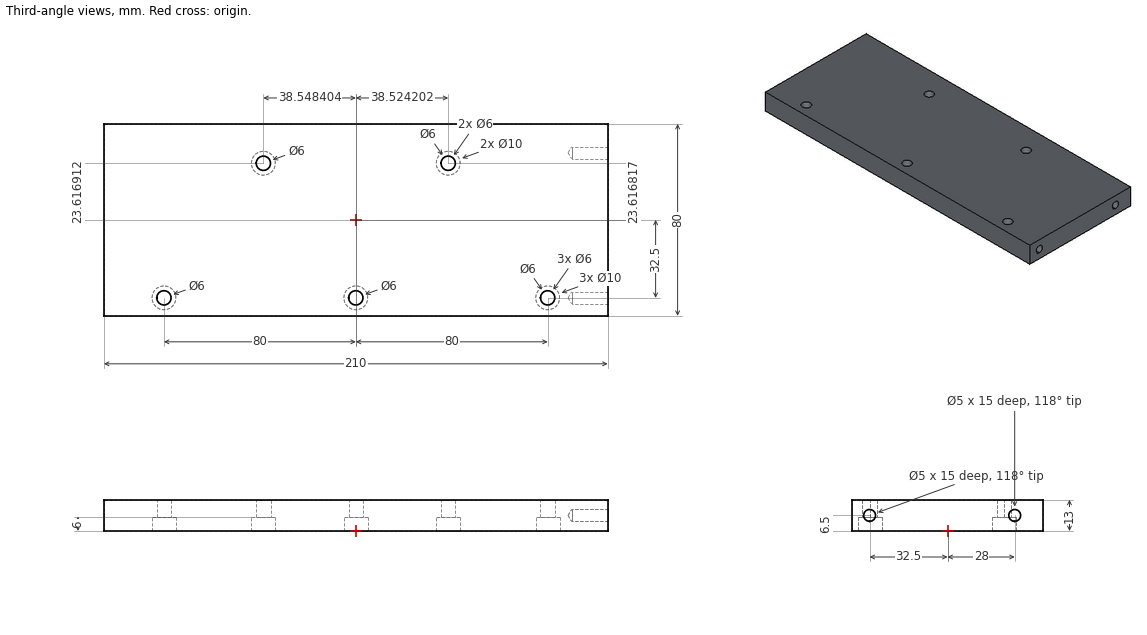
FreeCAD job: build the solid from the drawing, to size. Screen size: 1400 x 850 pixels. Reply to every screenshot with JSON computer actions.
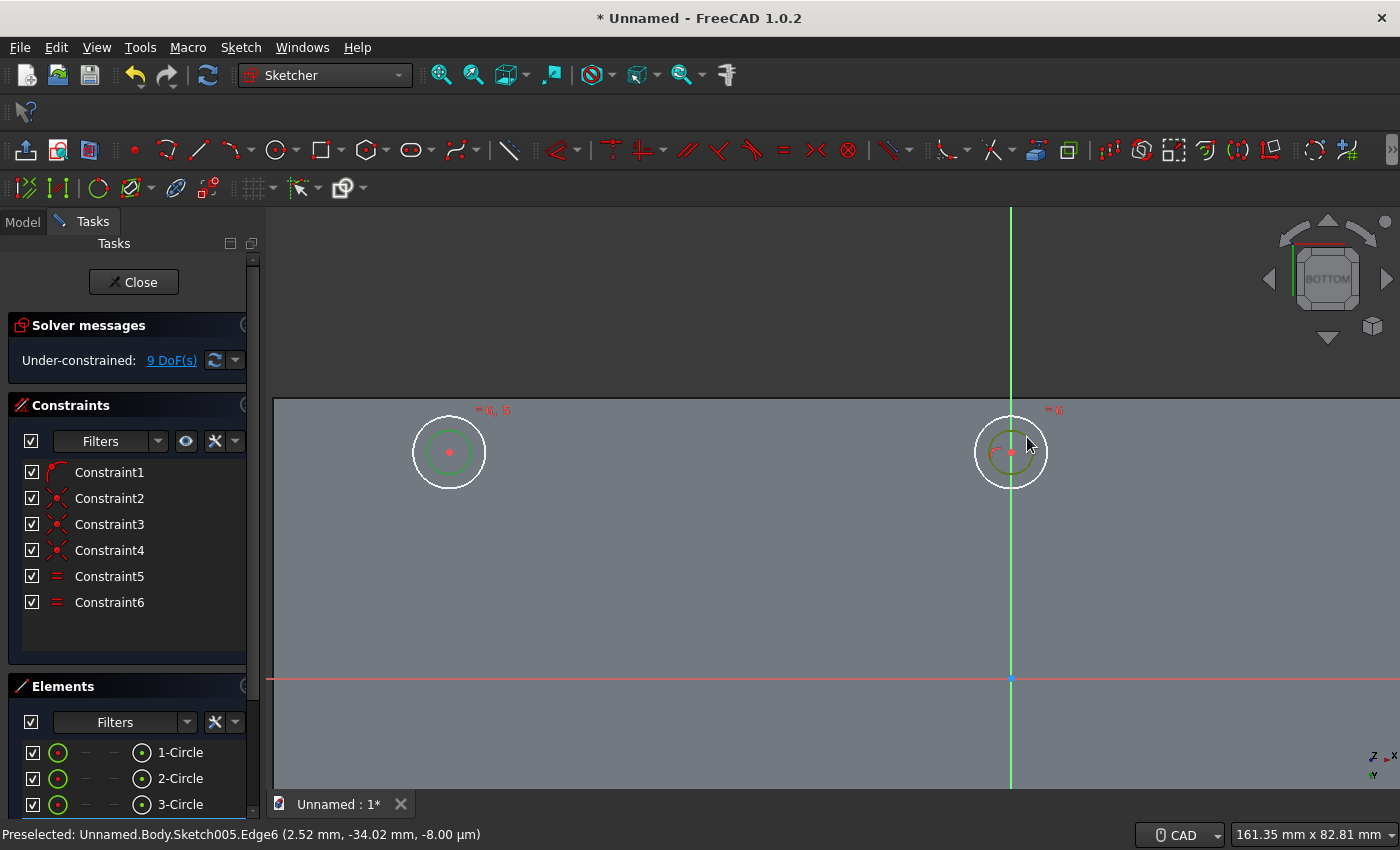
{"action": "left_click", "coordinate": [784, 150]}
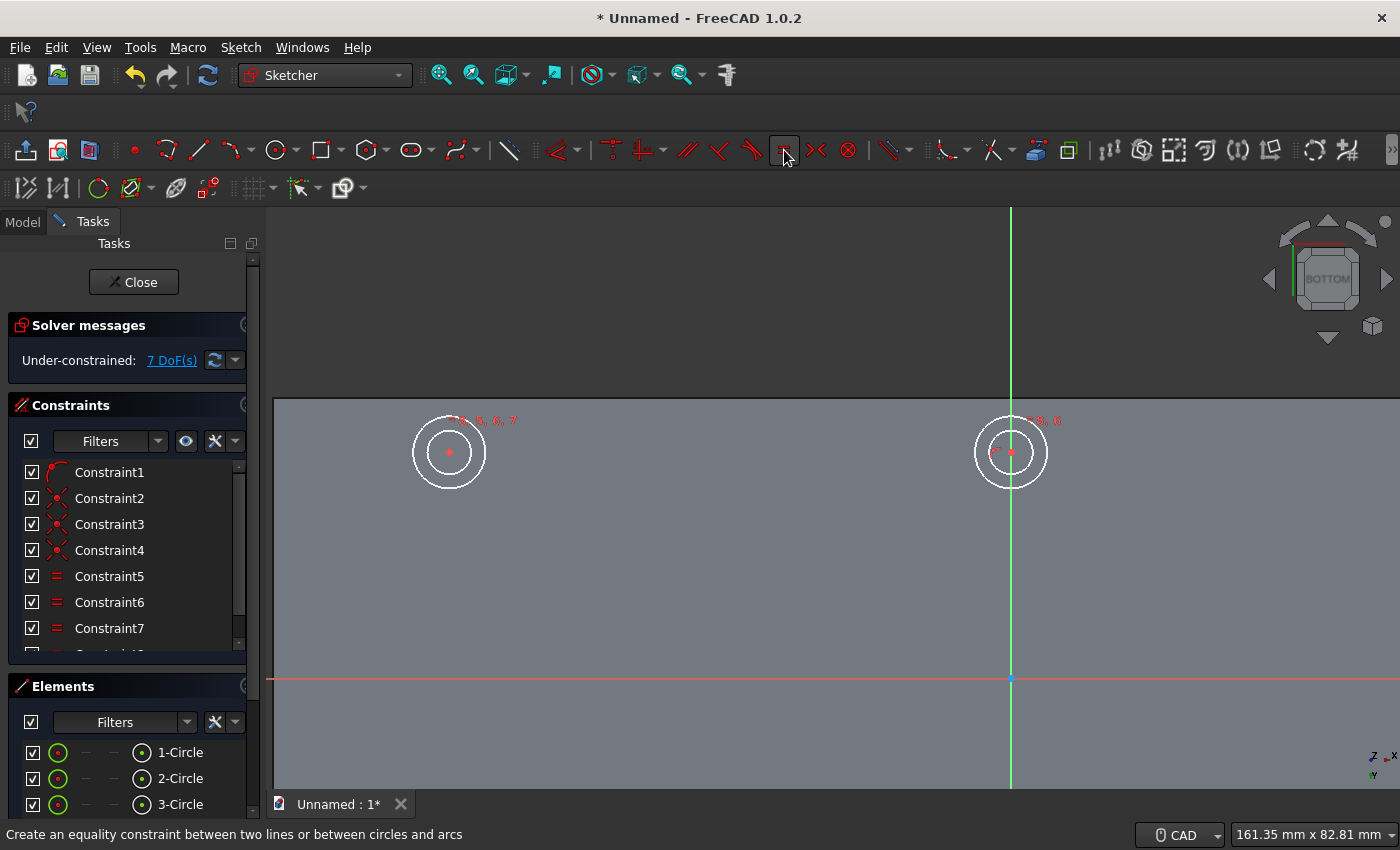
{"action": "scroll", "coordinate": [465, 438], "scroll_direction": "down", "scroll_amount": 3}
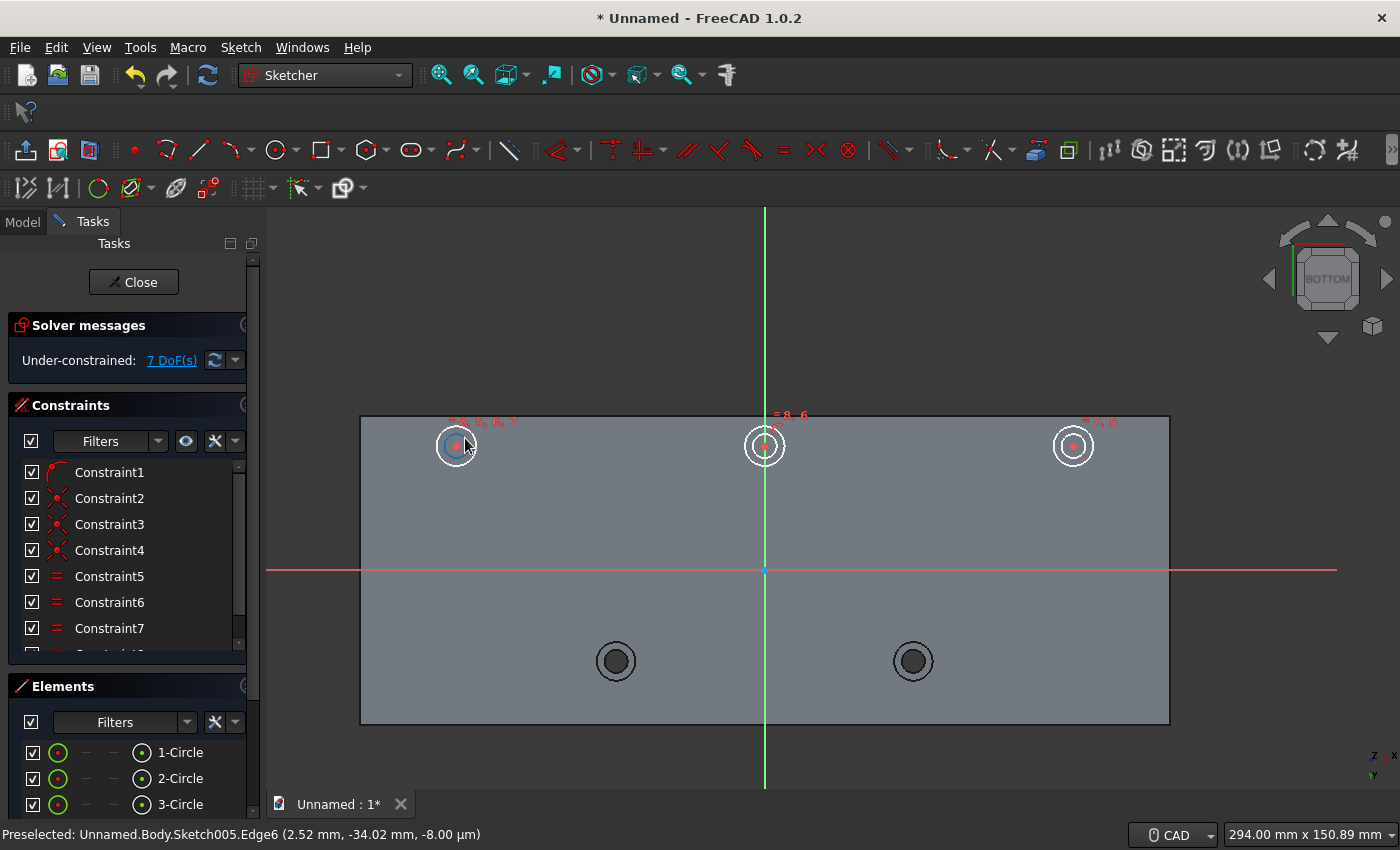
{"action": "left_click", "coordinate": [1073, 446]}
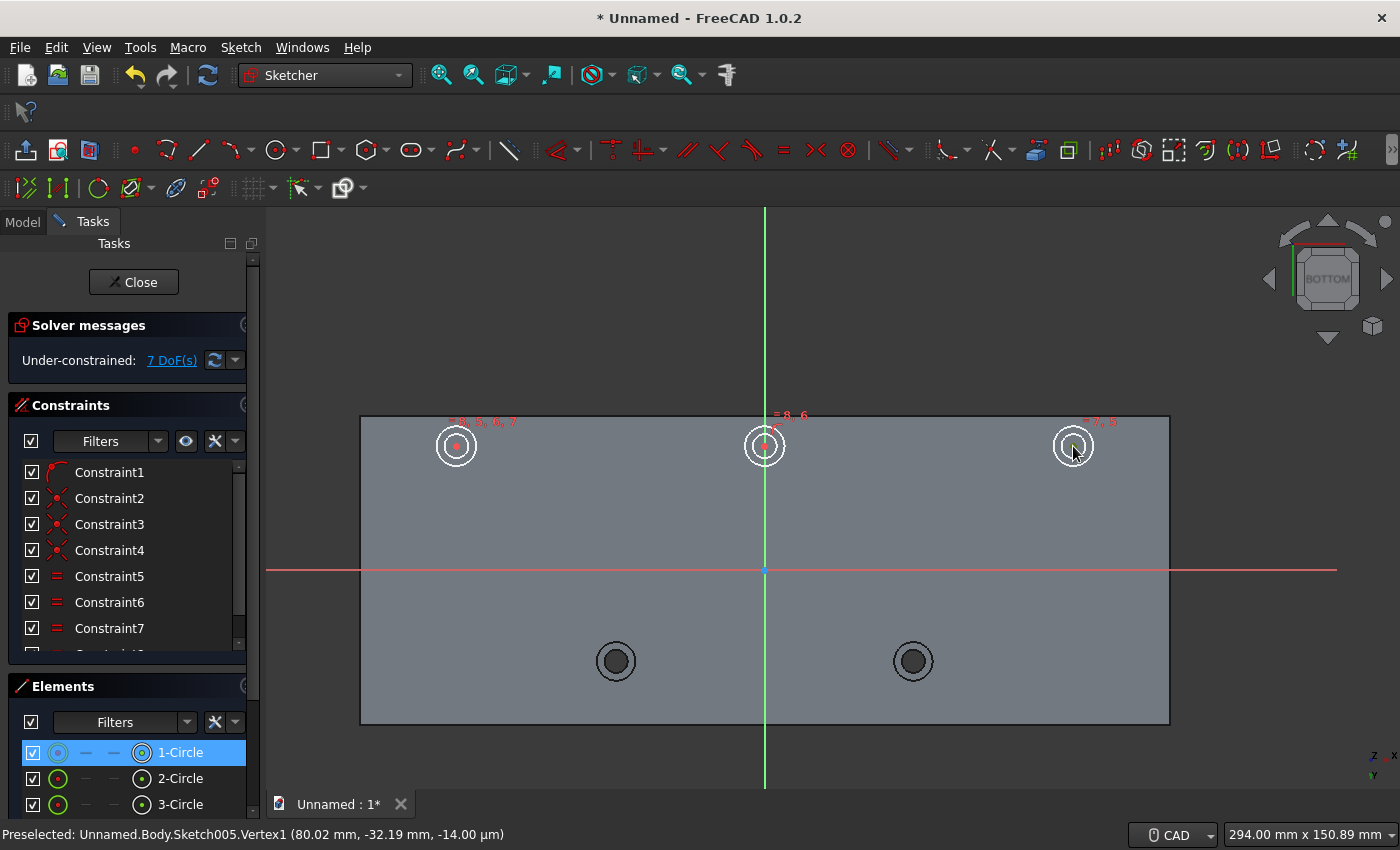
{"action": "left_click", "coordinate": [456, 446]}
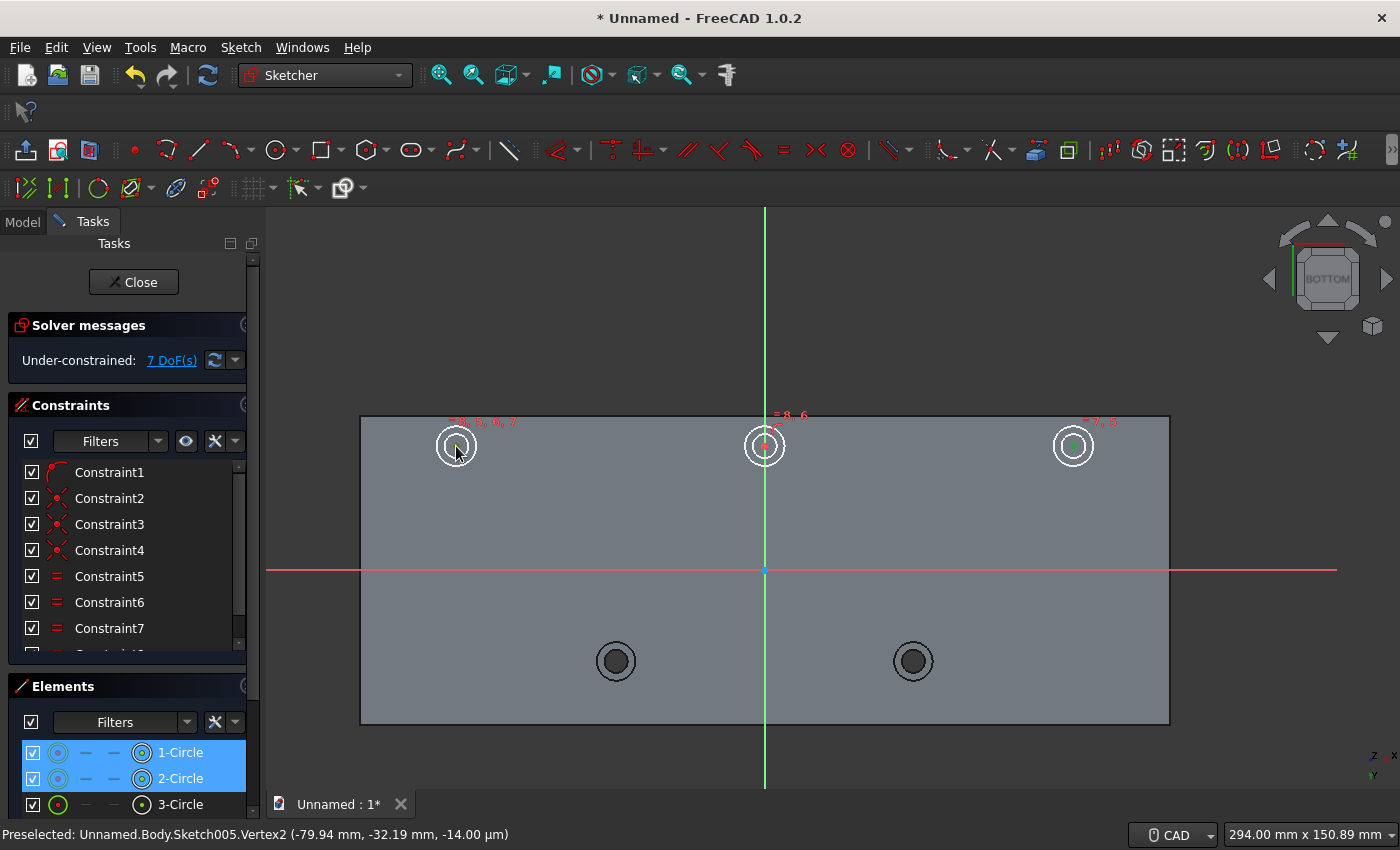
{"action": "key", "text": "h"}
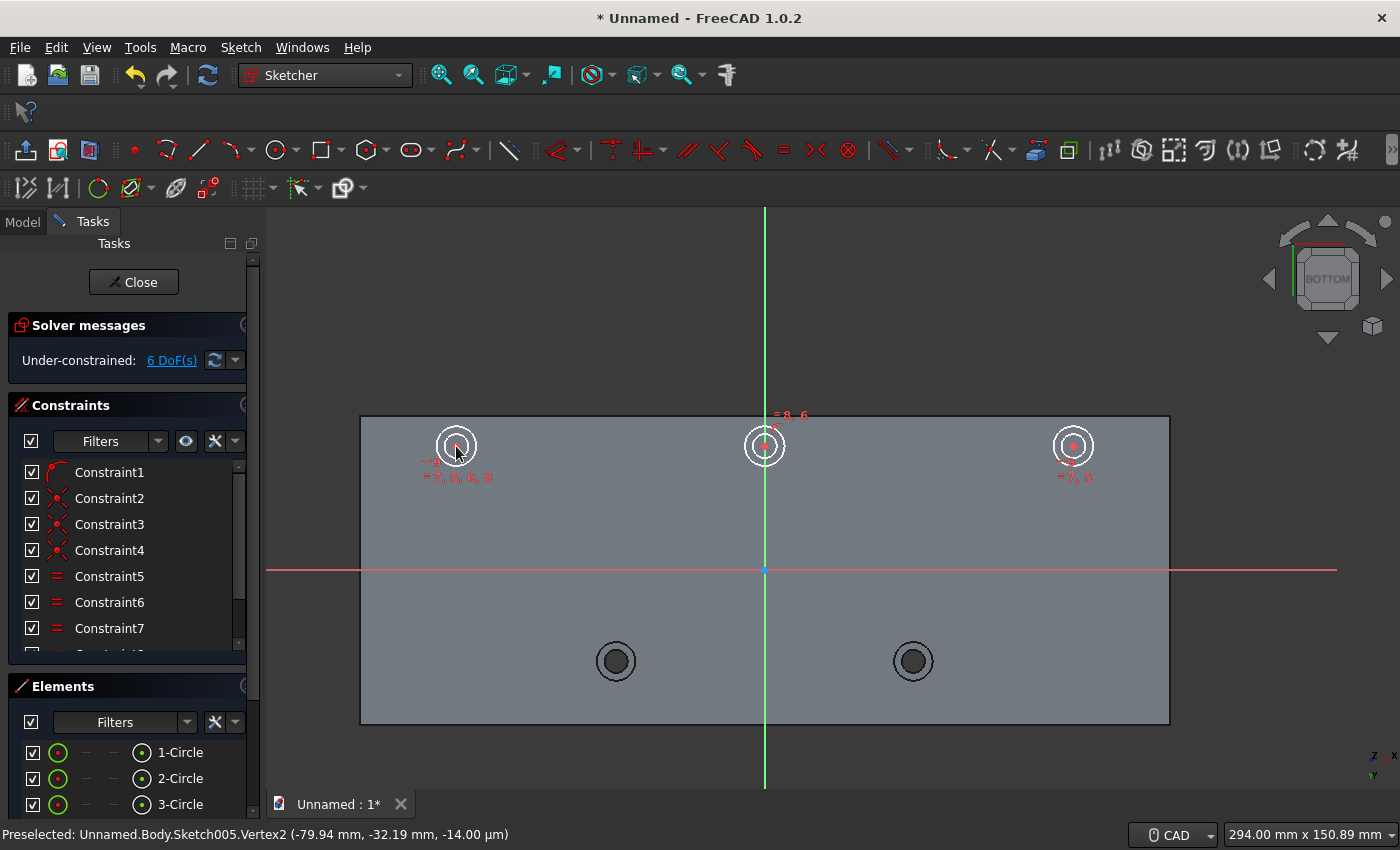
{"action": "left_click", "coordinate": [1073, 446]}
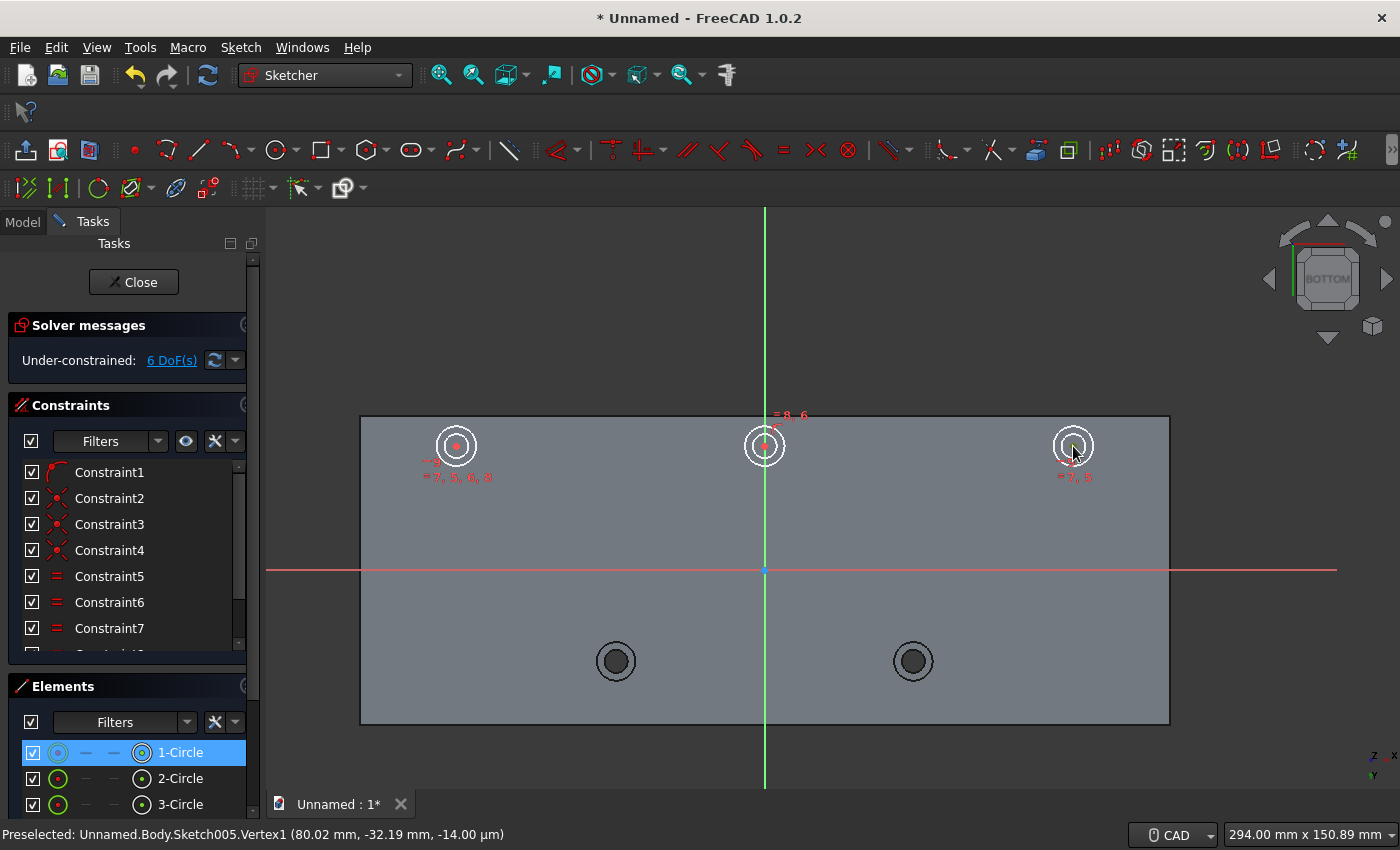
{"action": "left_click", "coordinate": [765, 446]}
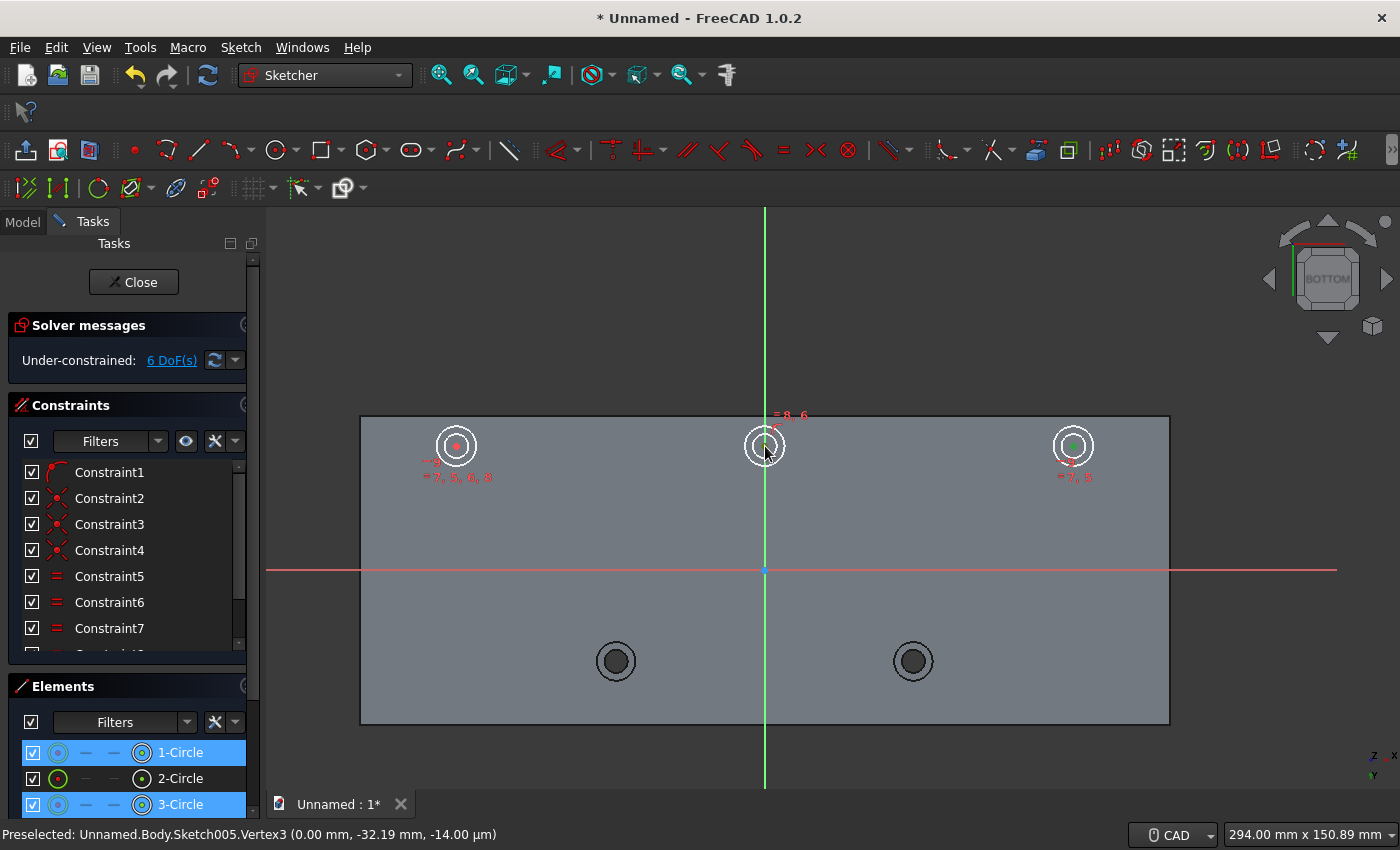
{"action": "left_click", "coordinate": [666, 150]}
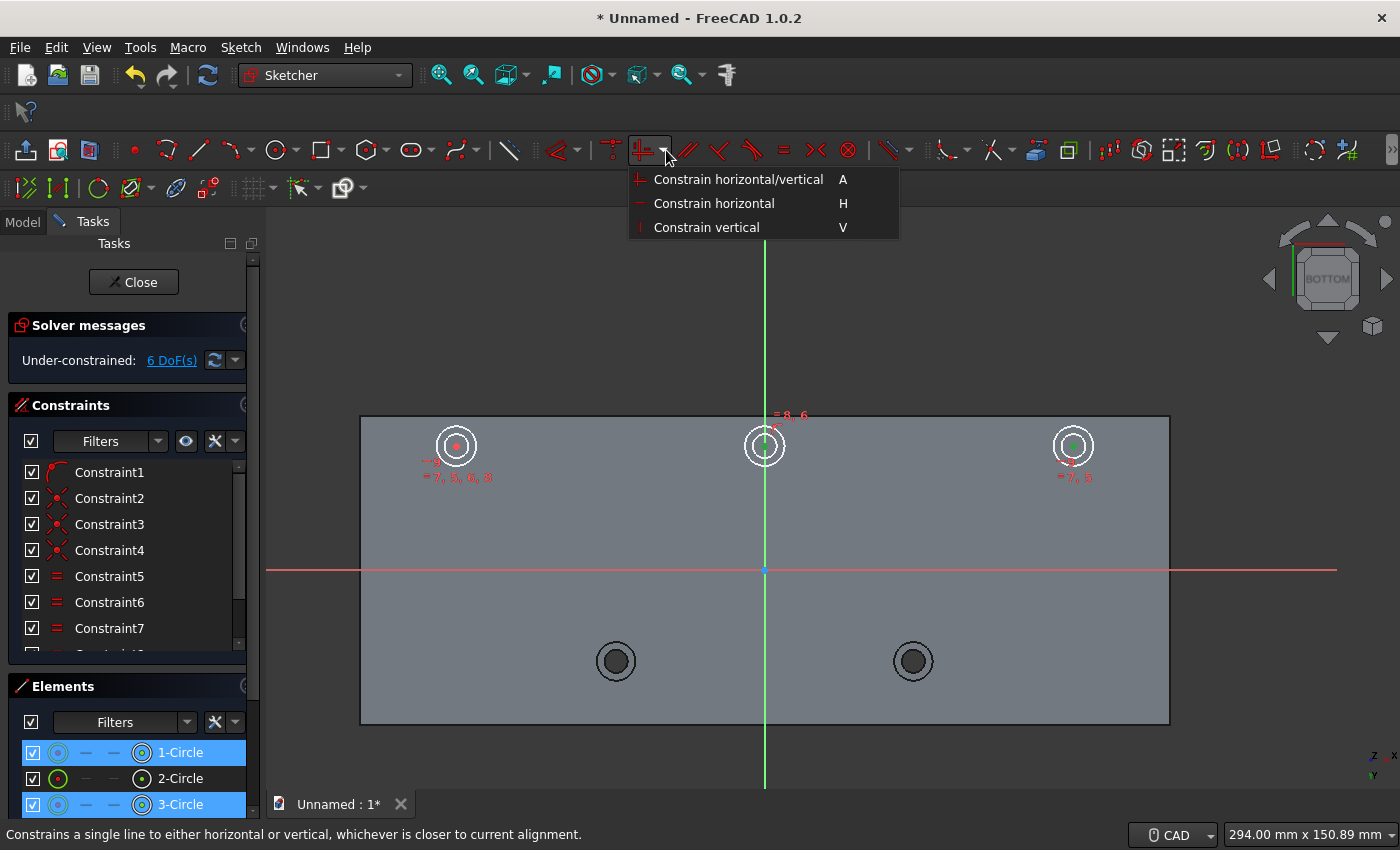
{"action": "left_click", "coordinate": [764, 203]}